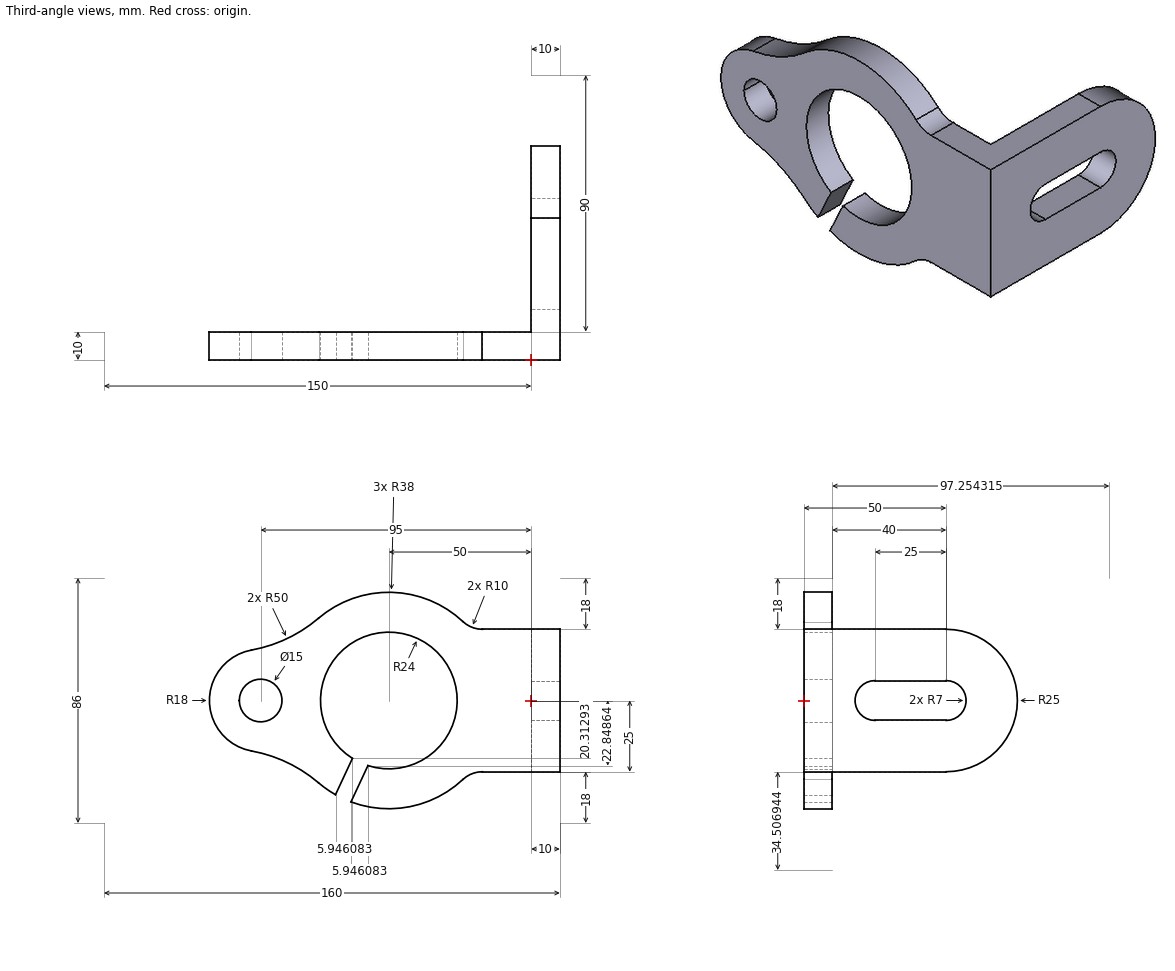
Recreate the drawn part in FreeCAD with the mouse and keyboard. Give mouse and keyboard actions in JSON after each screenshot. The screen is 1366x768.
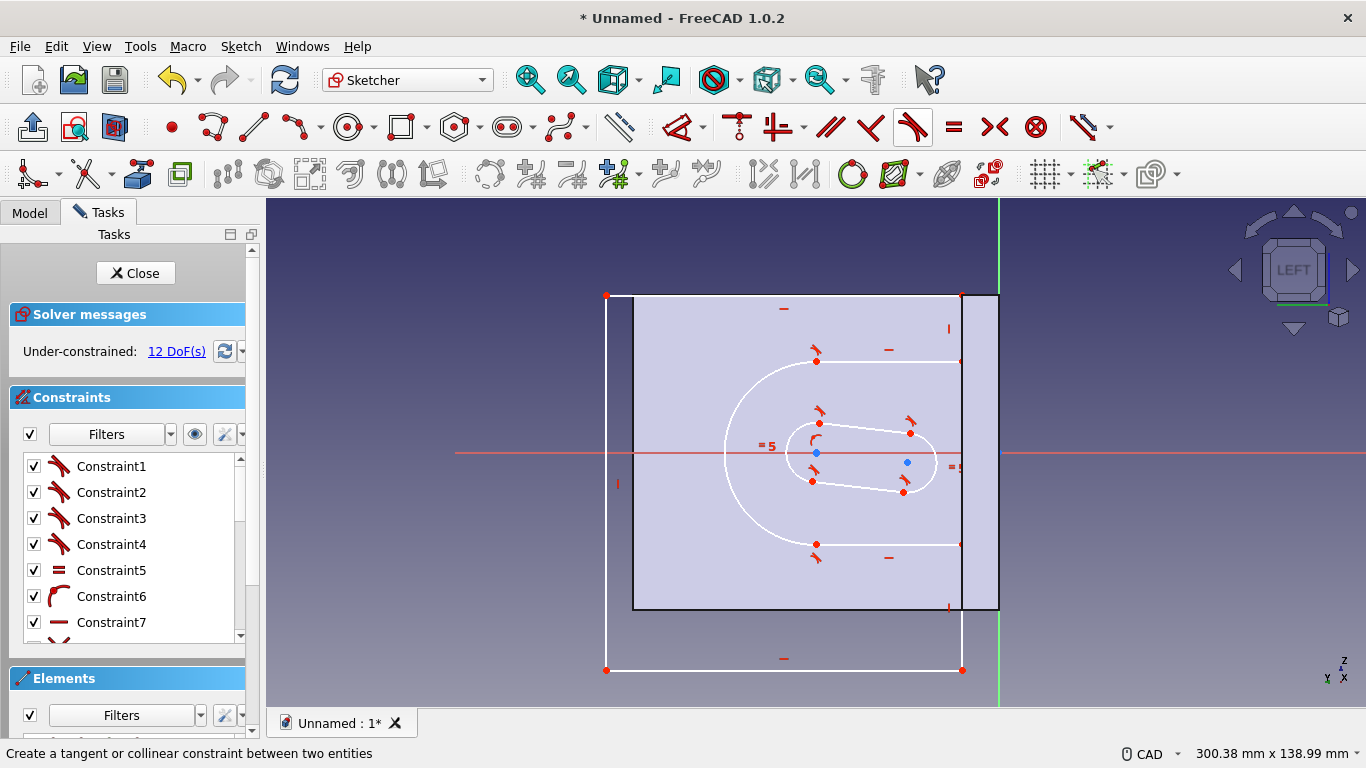
{"action": "left_click", "coordinate": [847, 426]}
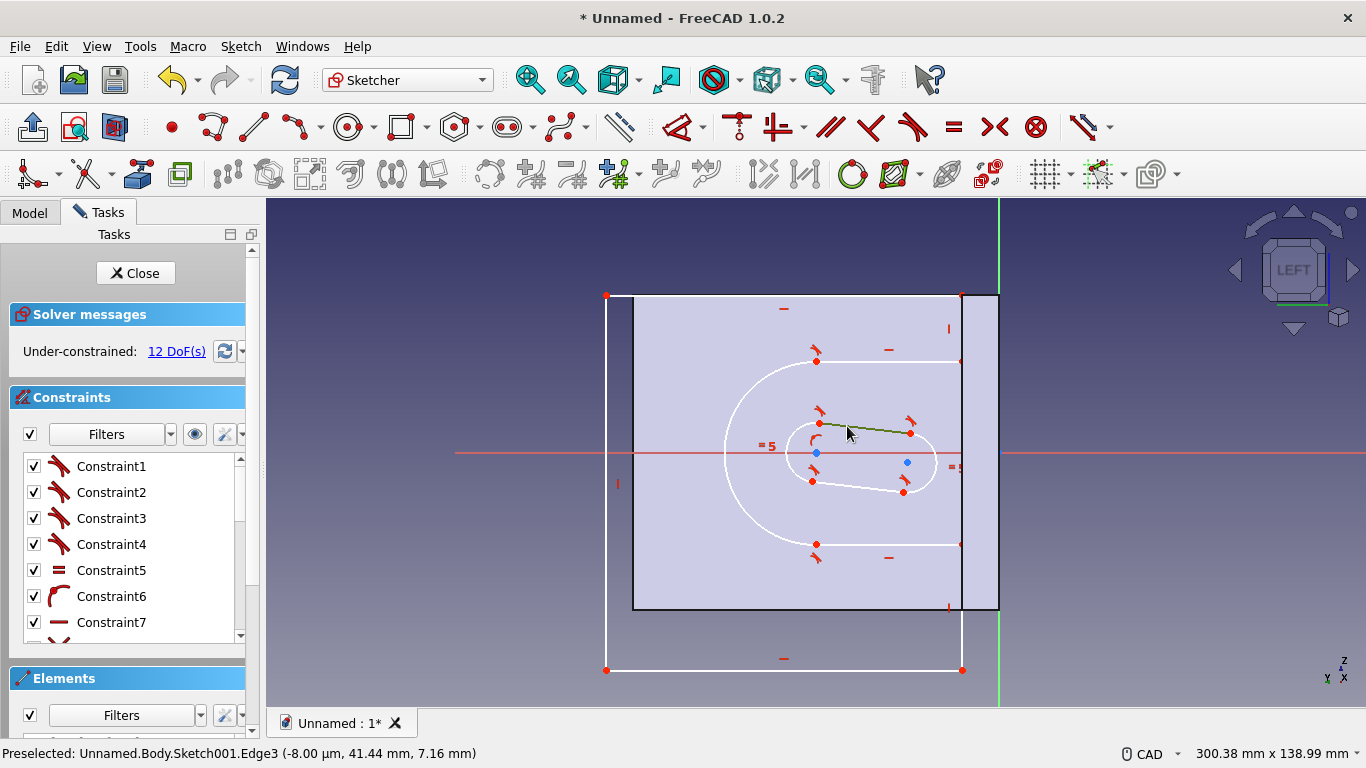
{"action": "key", "text": "h"}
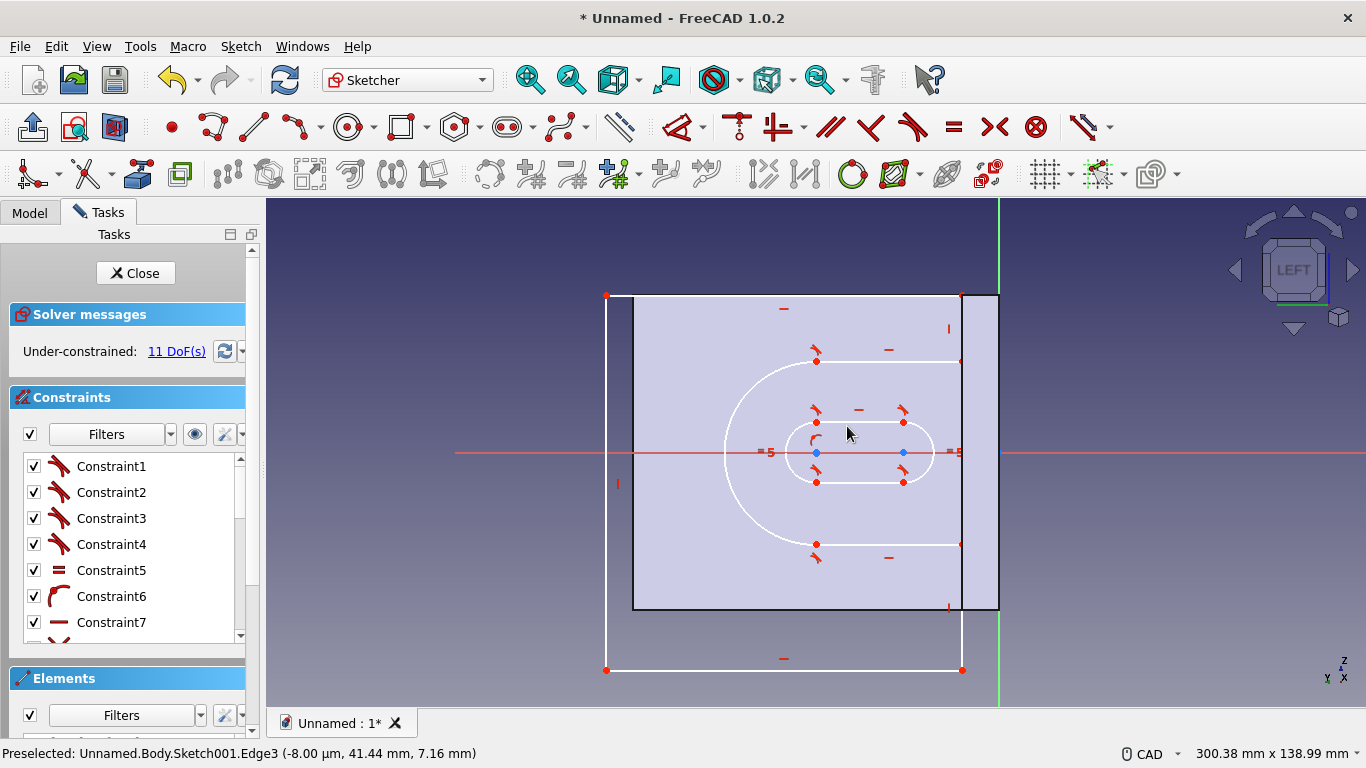
{"action": "left_click", "coordinate": [792, 435]}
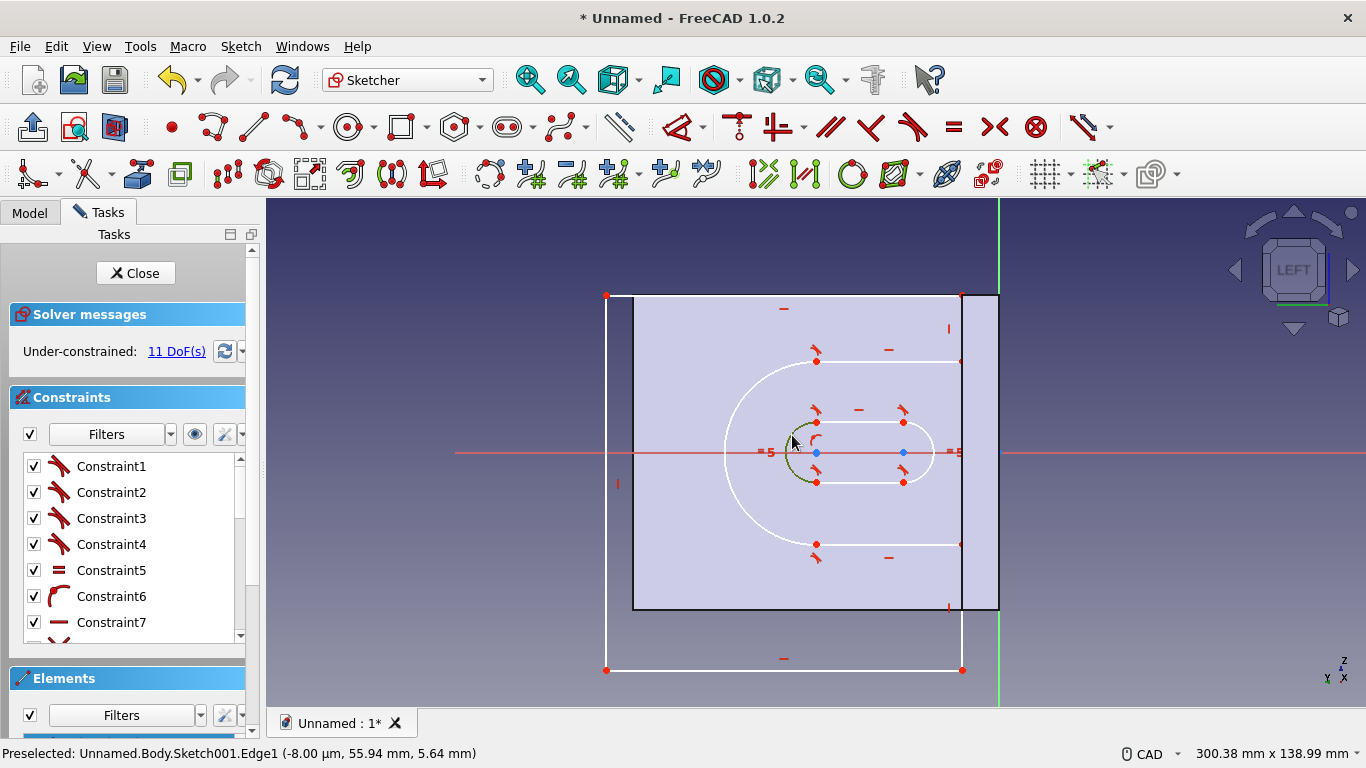
{"action": "left_click", "coordinate": [742, 400]}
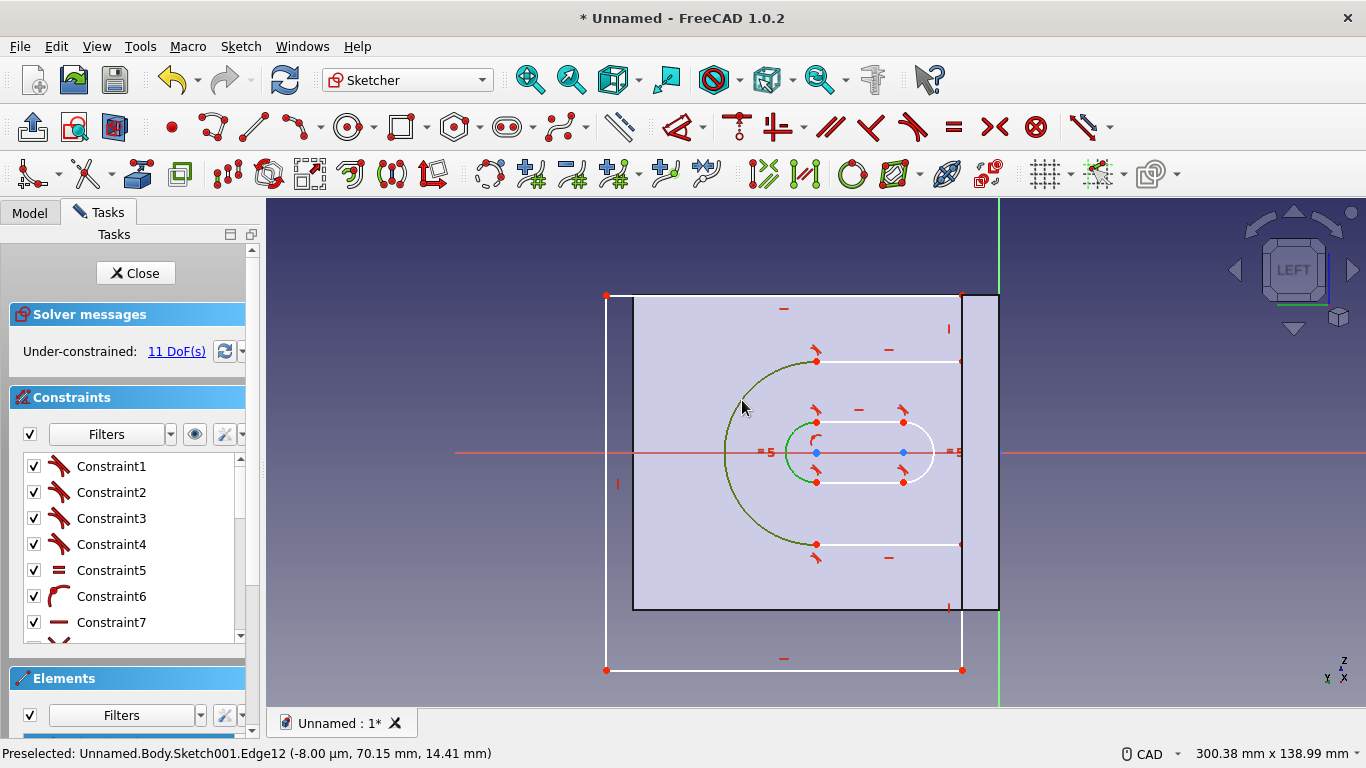
{"action": "key", "text": "c"}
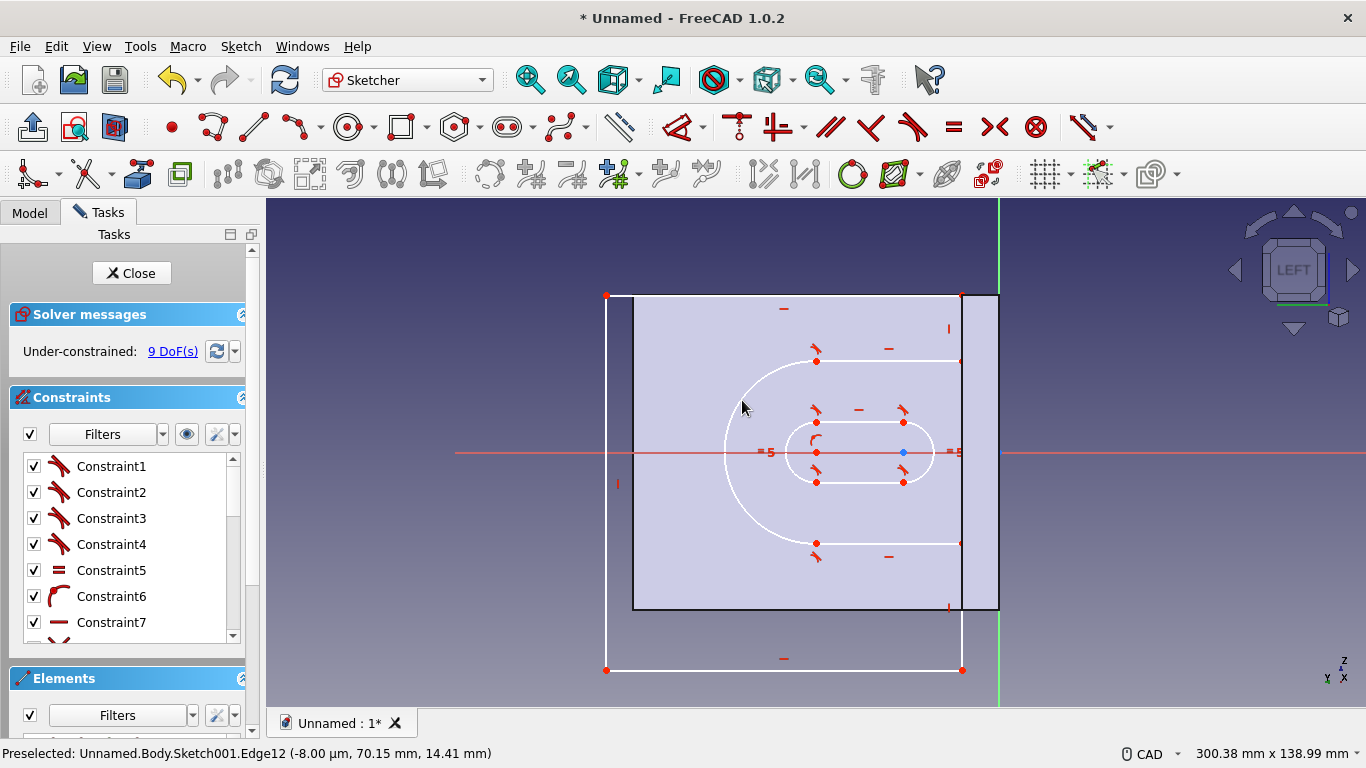
{"action": "scroll", "coordinate": [792, 435], "scroll_direction": "up", "scroll_amount": 3}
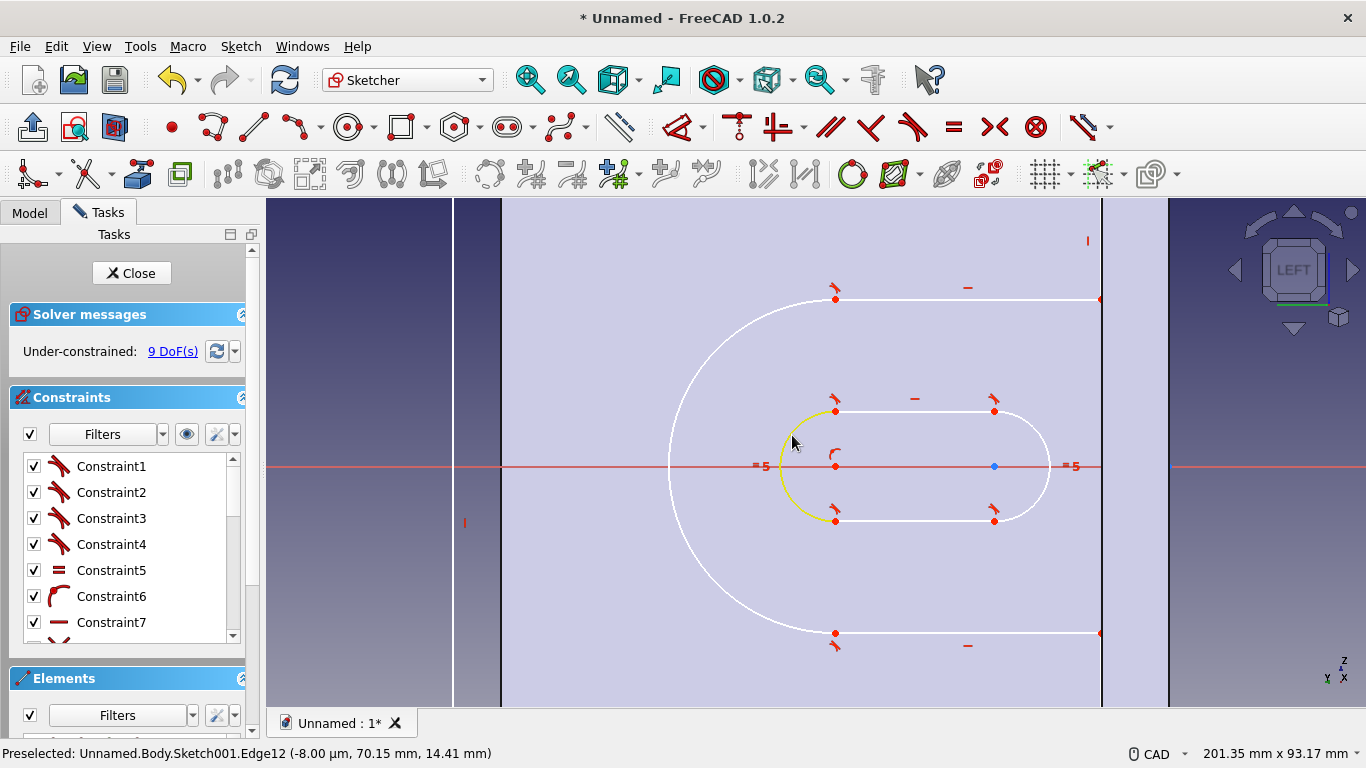
{"action": "left_click", "coordinate": [791, 434]}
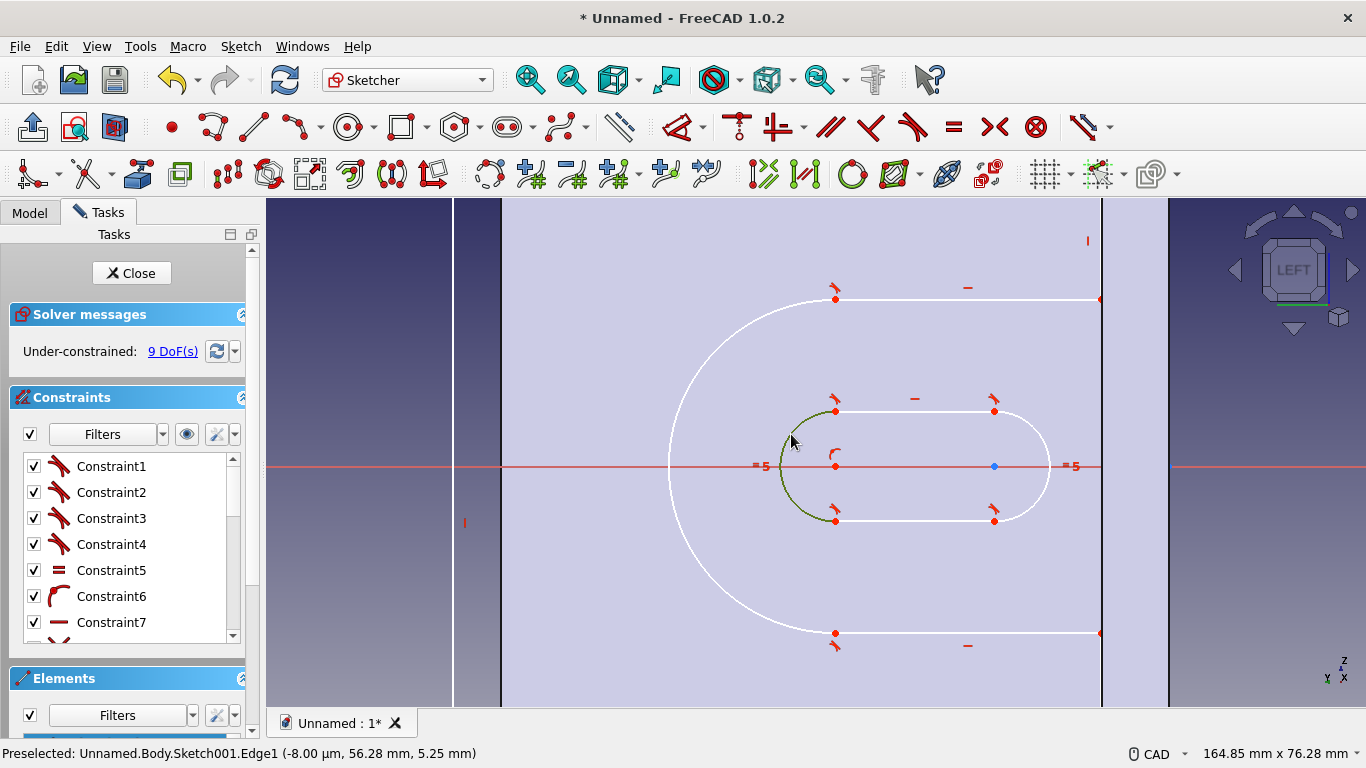
{"action": "left_click", "coordinate": [702, 128]}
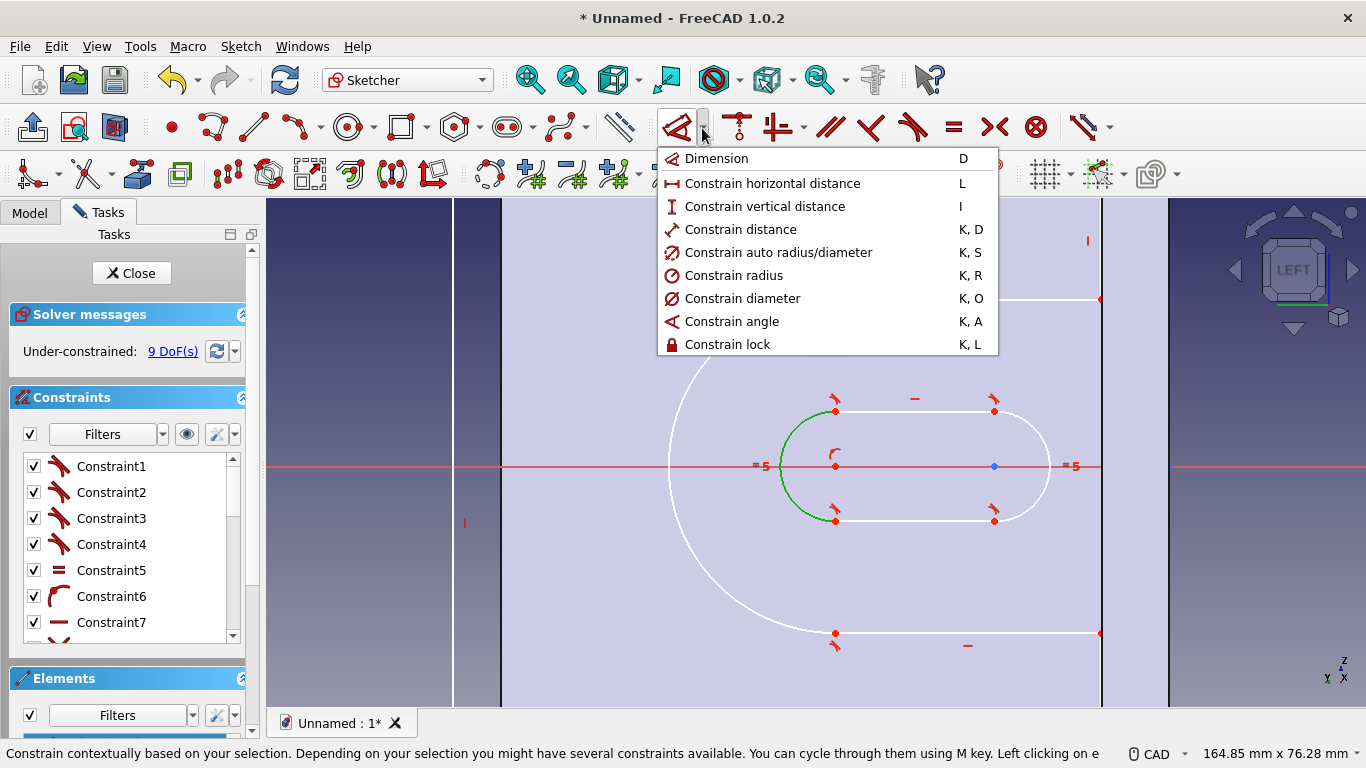
{"action": "left_click", "coordinate": [828, 276]}